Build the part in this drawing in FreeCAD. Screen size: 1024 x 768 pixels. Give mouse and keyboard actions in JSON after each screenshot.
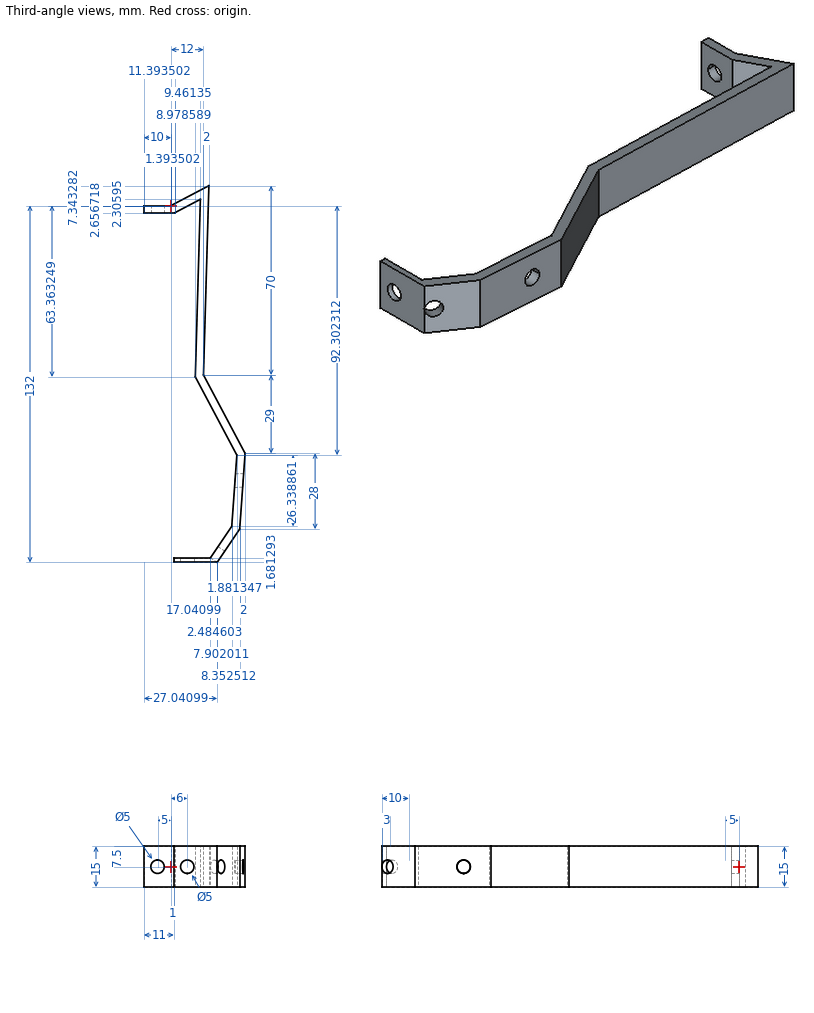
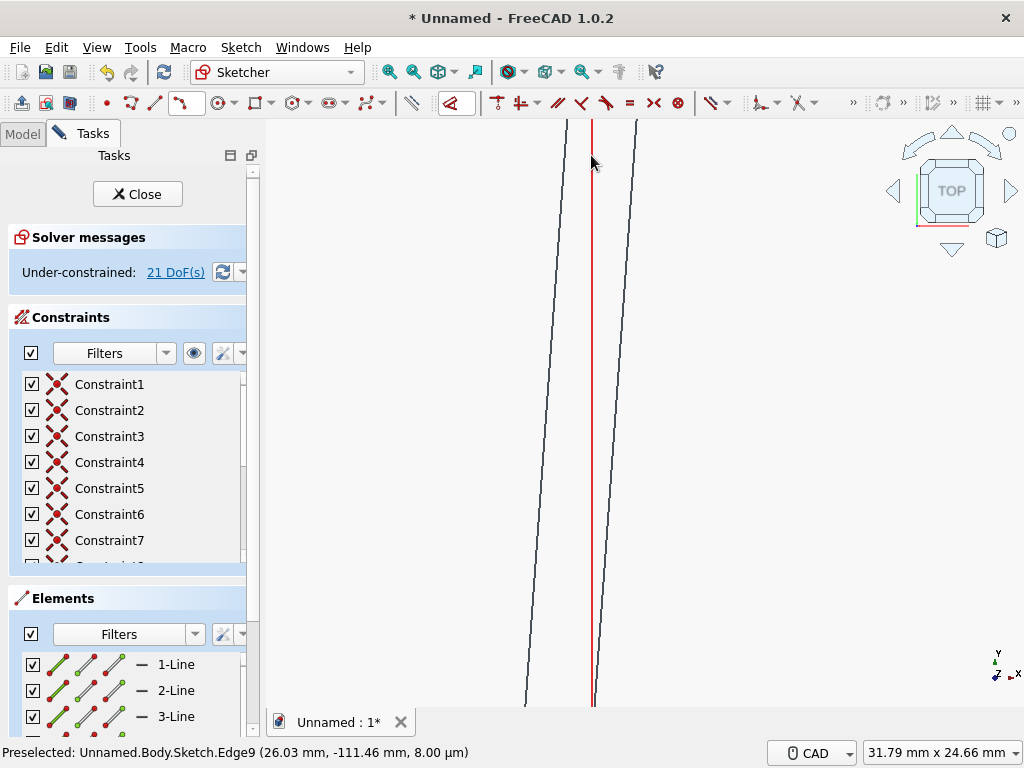
{"action": "scroll", "coordinate": [609, 543], "scroll_direction": "down", "scroll_amount": 11}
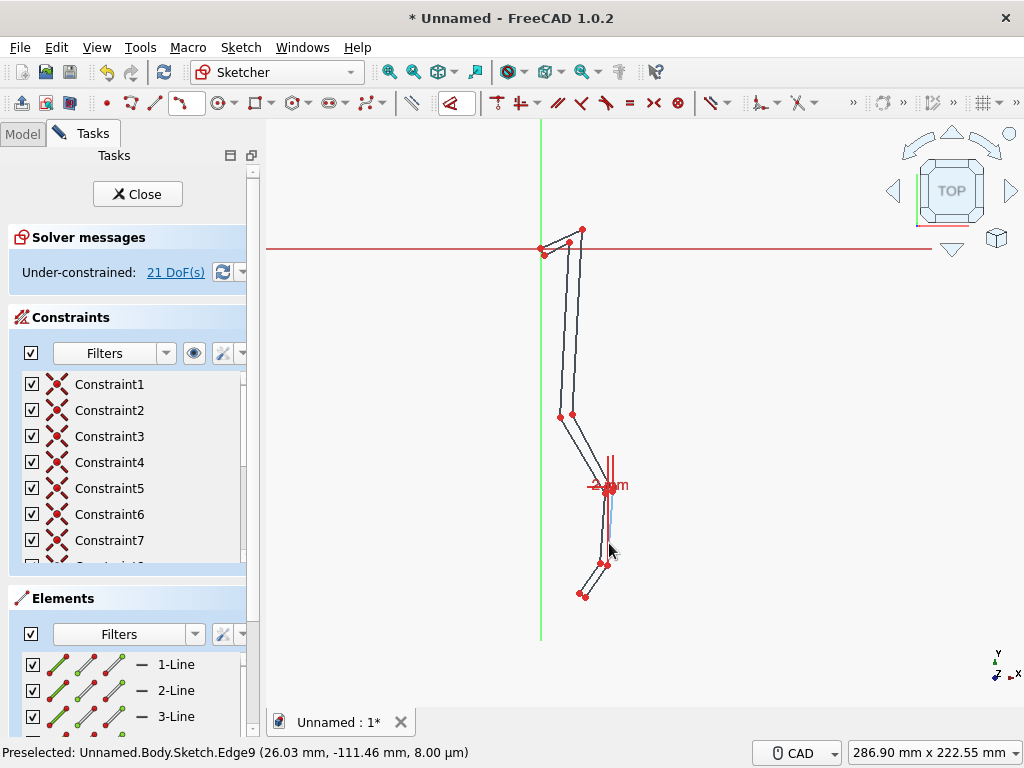
{"action": "scroll", "coordinate": [575, 359], "scroll_direction": "up", "scroll_amount": 11}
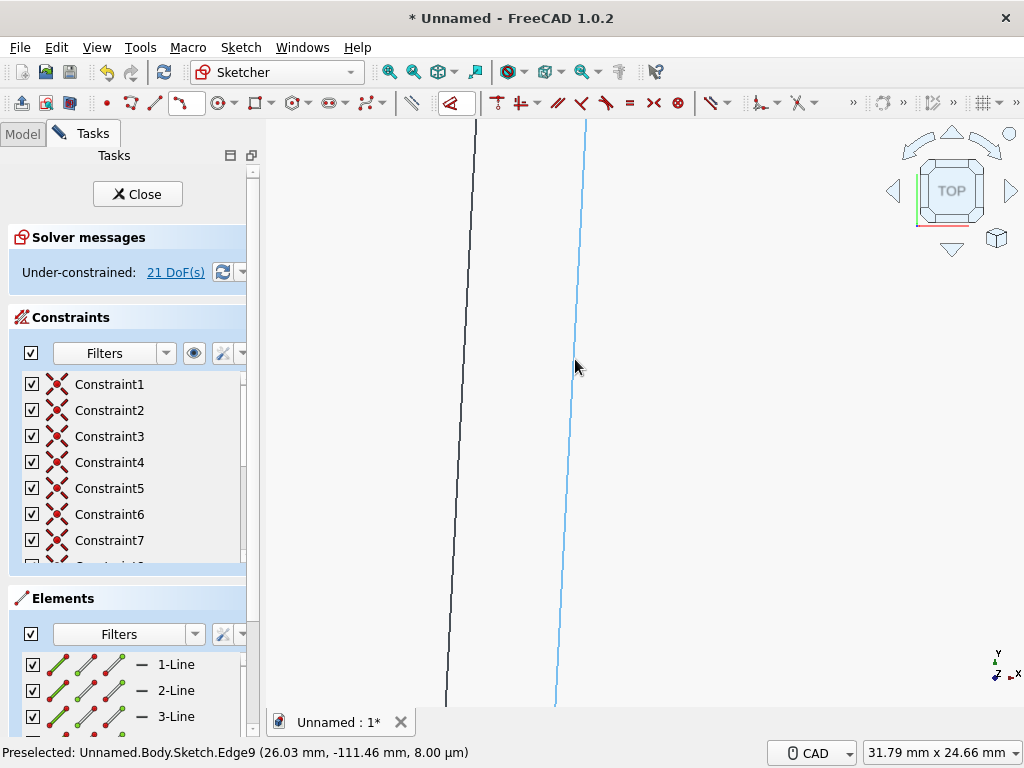
{"action": "left_click", "coordinate": [574, 358]}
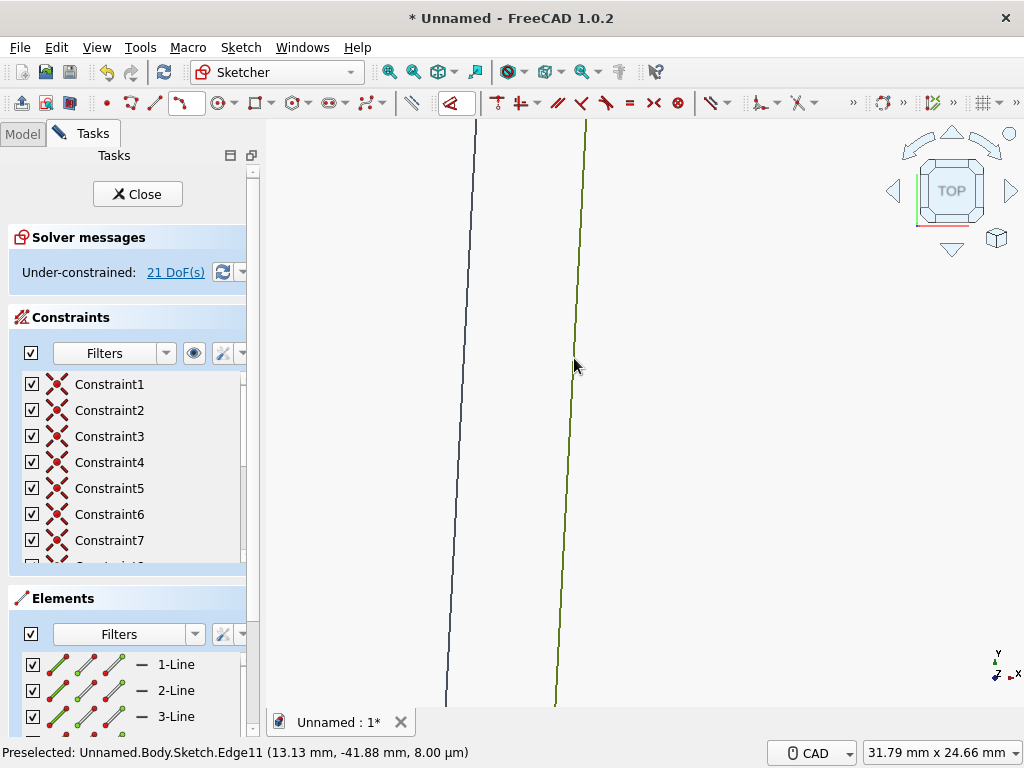
{"action": "left_click", "coordinate": [470, 104]}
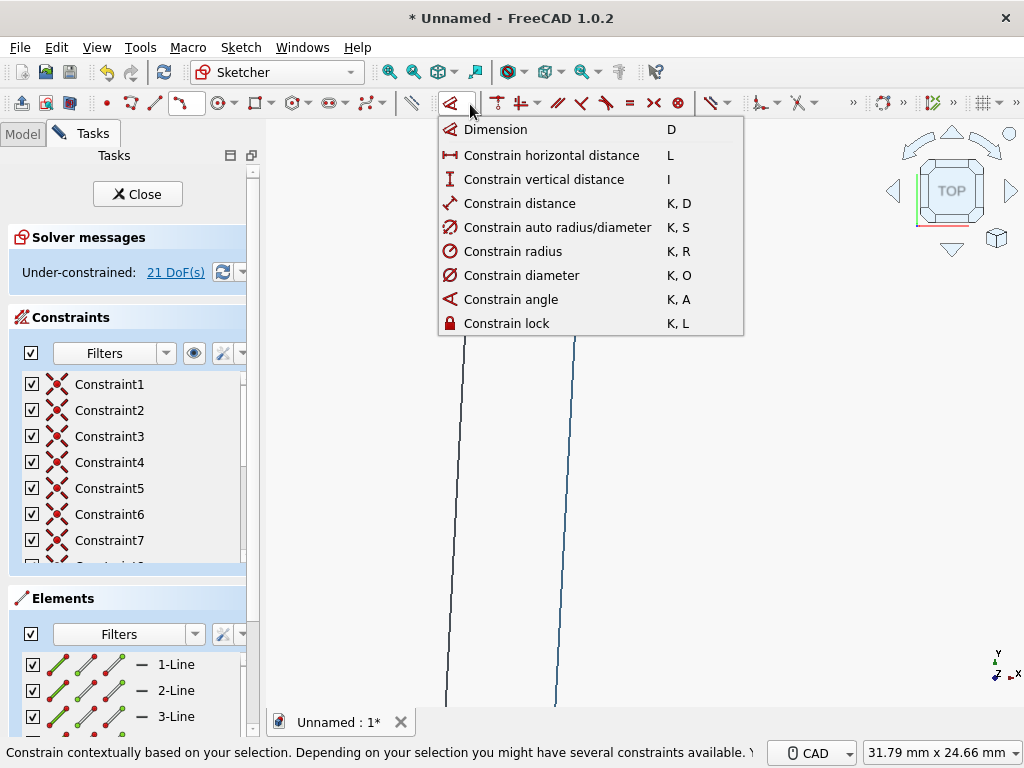
{"action": "left_click", "coordinate": [591, 155]}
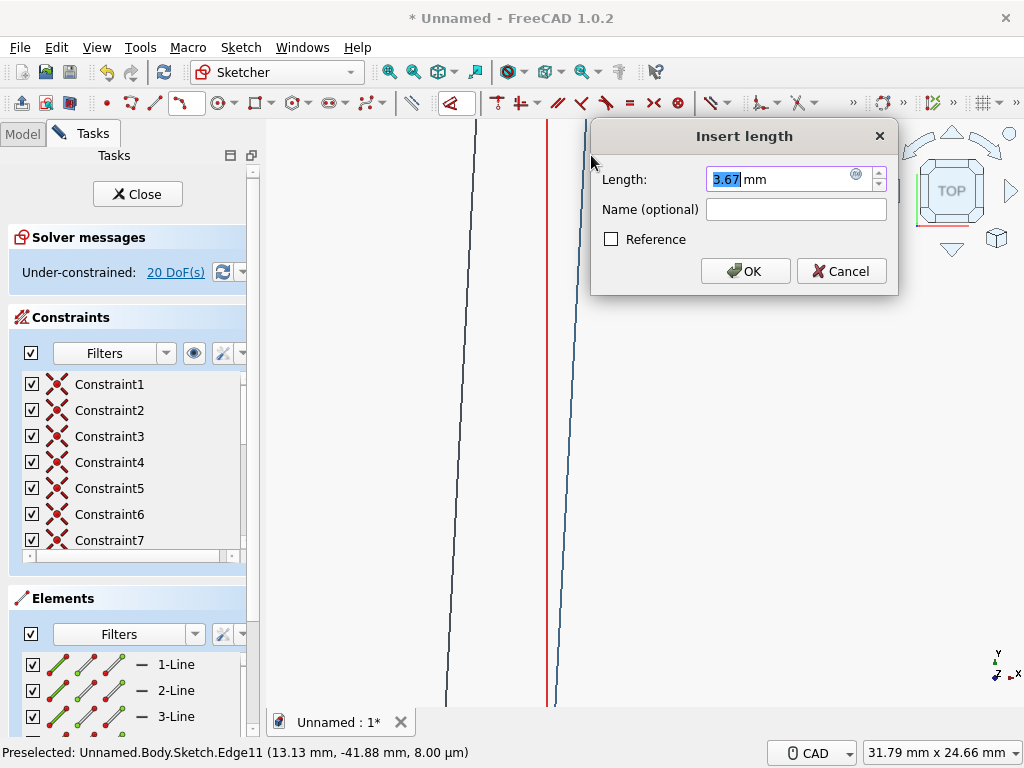
{"action": "type", "text": "2"}
{"action": "key", "text": "Return"}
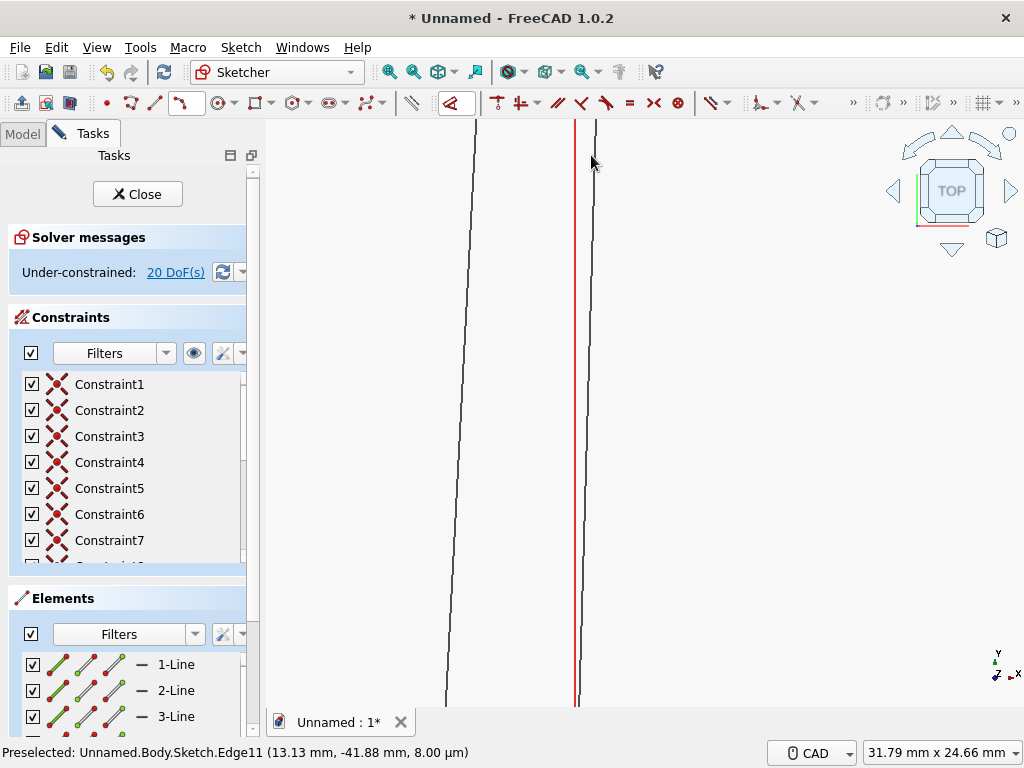
{"action": "scroll", "coordinate": [575, 359], "scroll_direction": "down", "scroll_amount": 11}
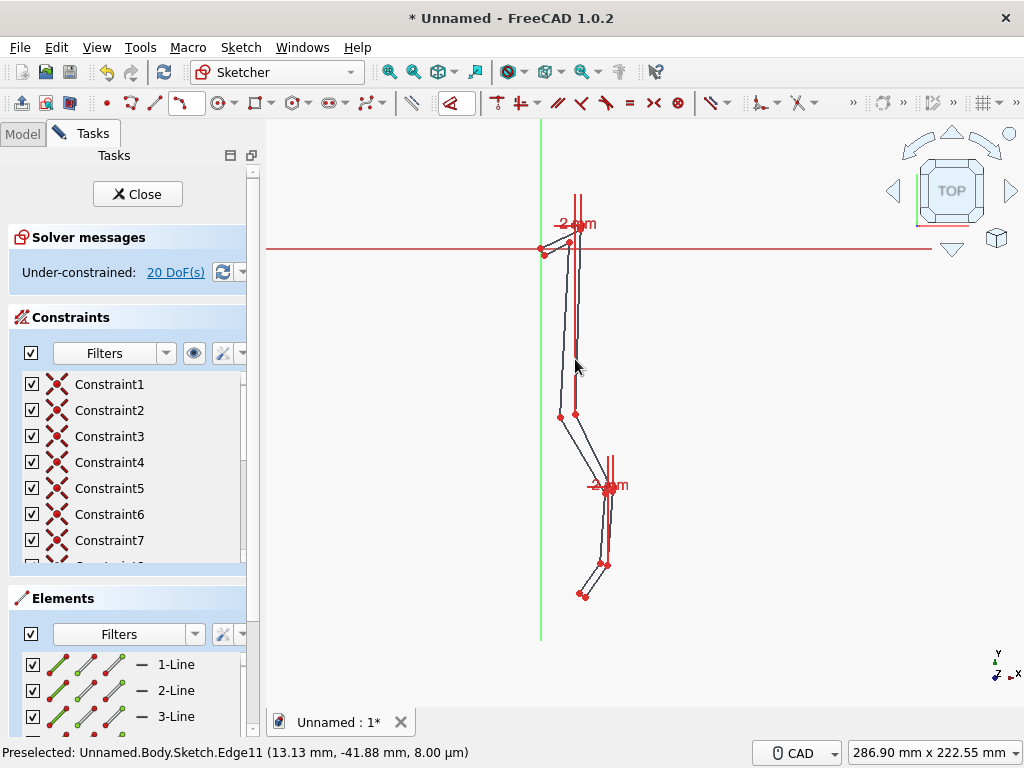
{"action": "scroll", "coordinate": [575, 415], "scroll_direction": "up", "scroll_amount": 2}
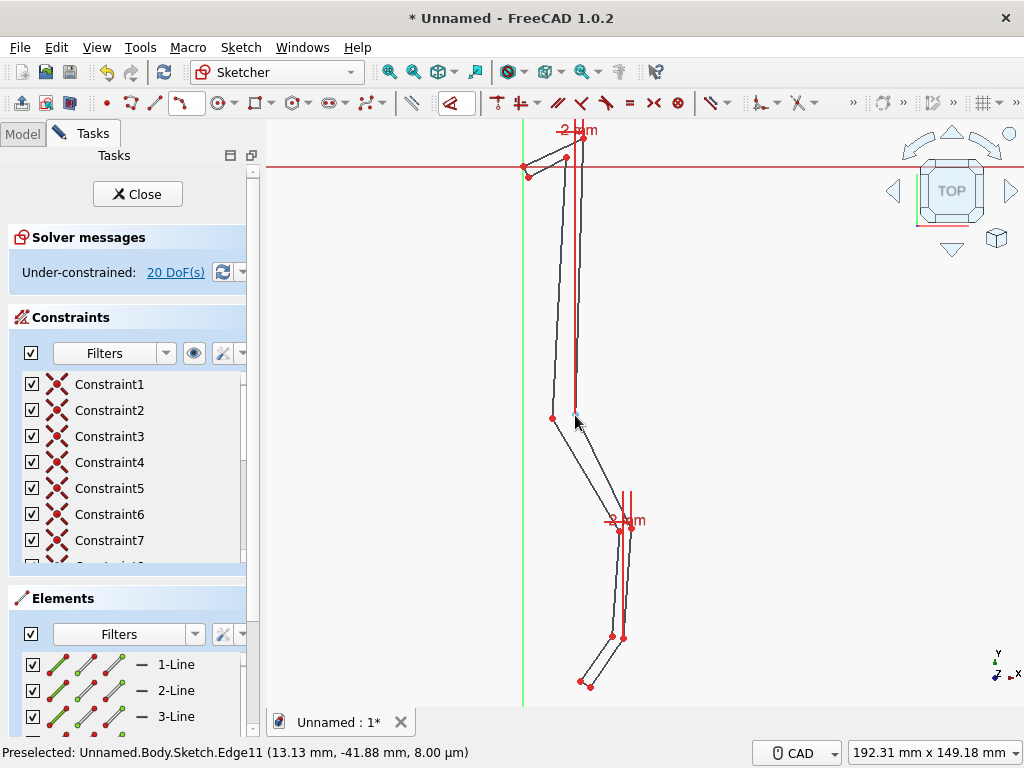
{"action": "left_click", "coordinate": [575, 414]}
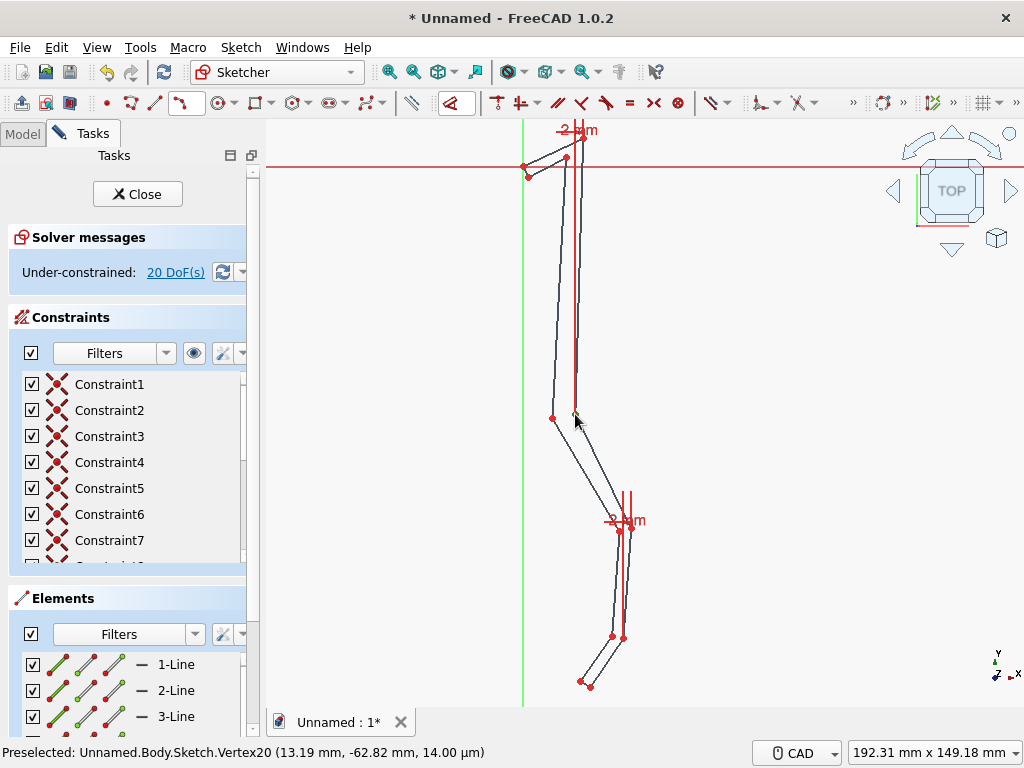
{"action": "key", "text": "l"}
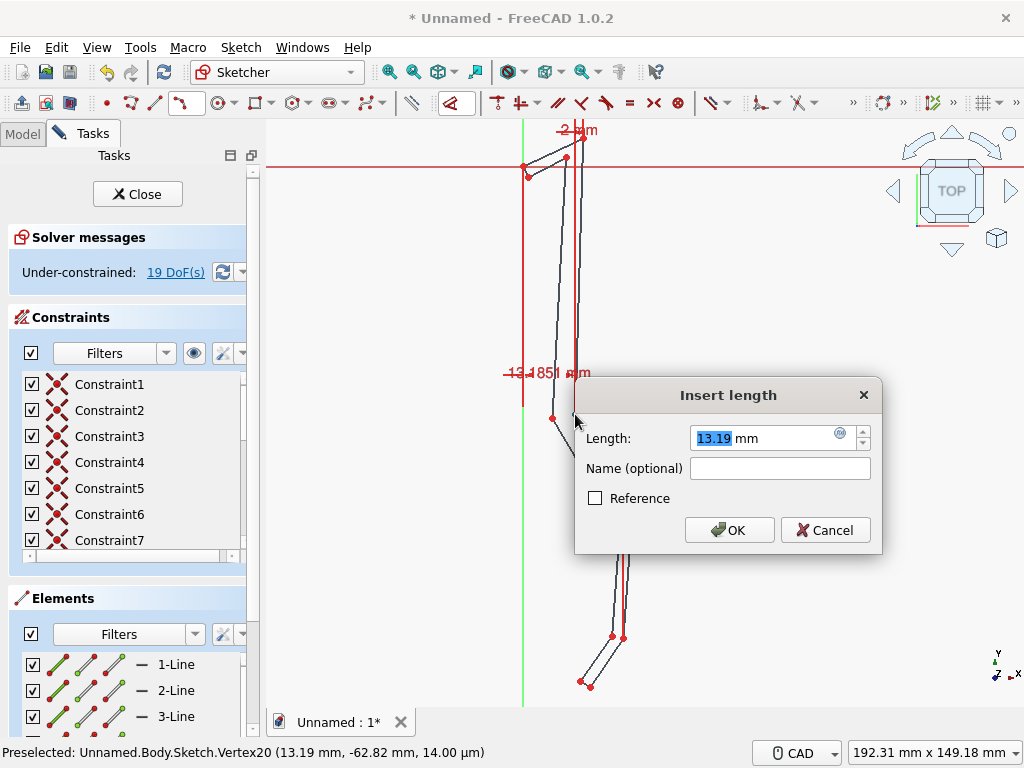
{"action": "type", "text": "12"}
{"action": "key", "text": "Return"}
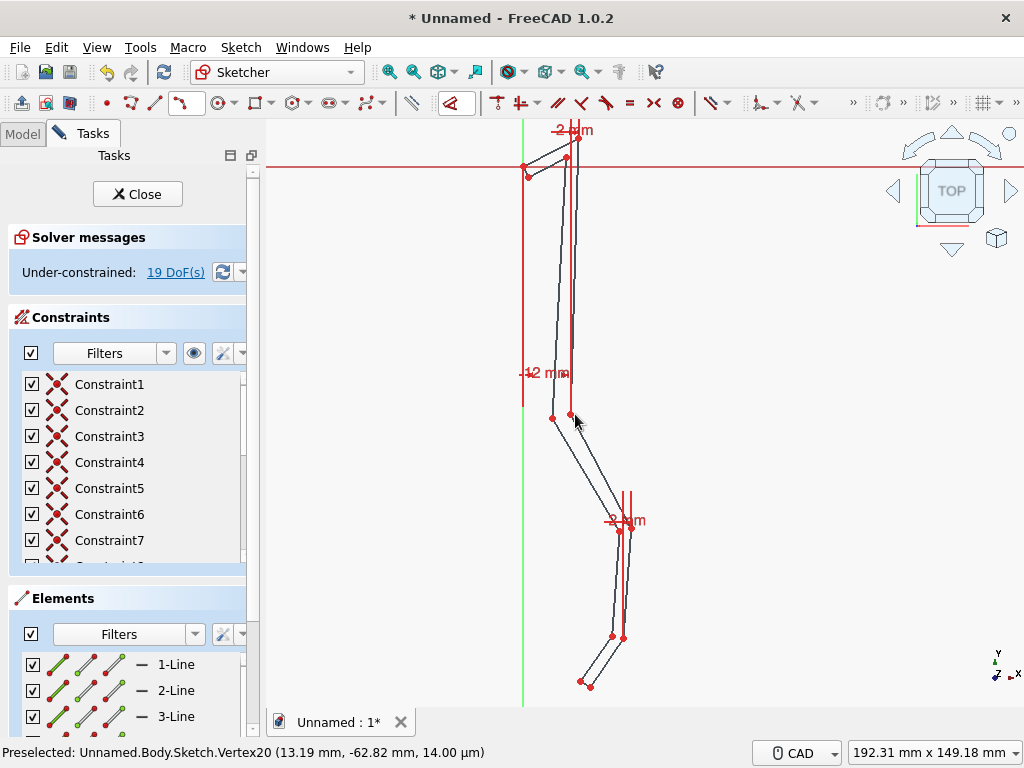
{"action": "left_click", "coordinate": [626, 606]}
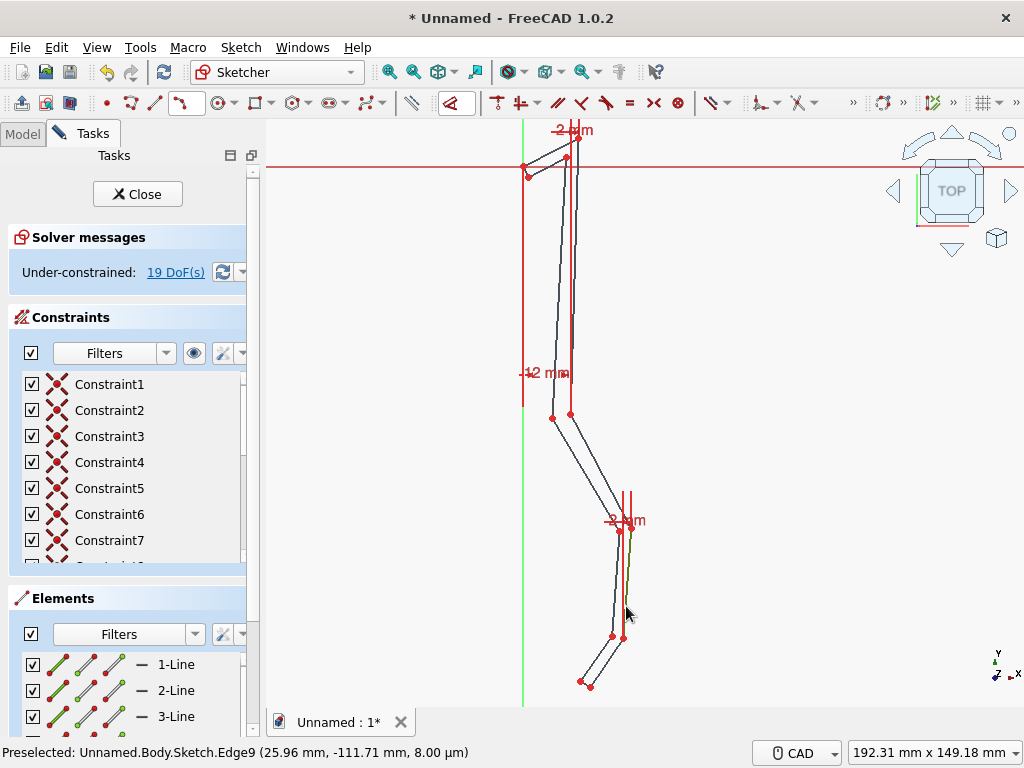
{"action": "key", "text": "i"}